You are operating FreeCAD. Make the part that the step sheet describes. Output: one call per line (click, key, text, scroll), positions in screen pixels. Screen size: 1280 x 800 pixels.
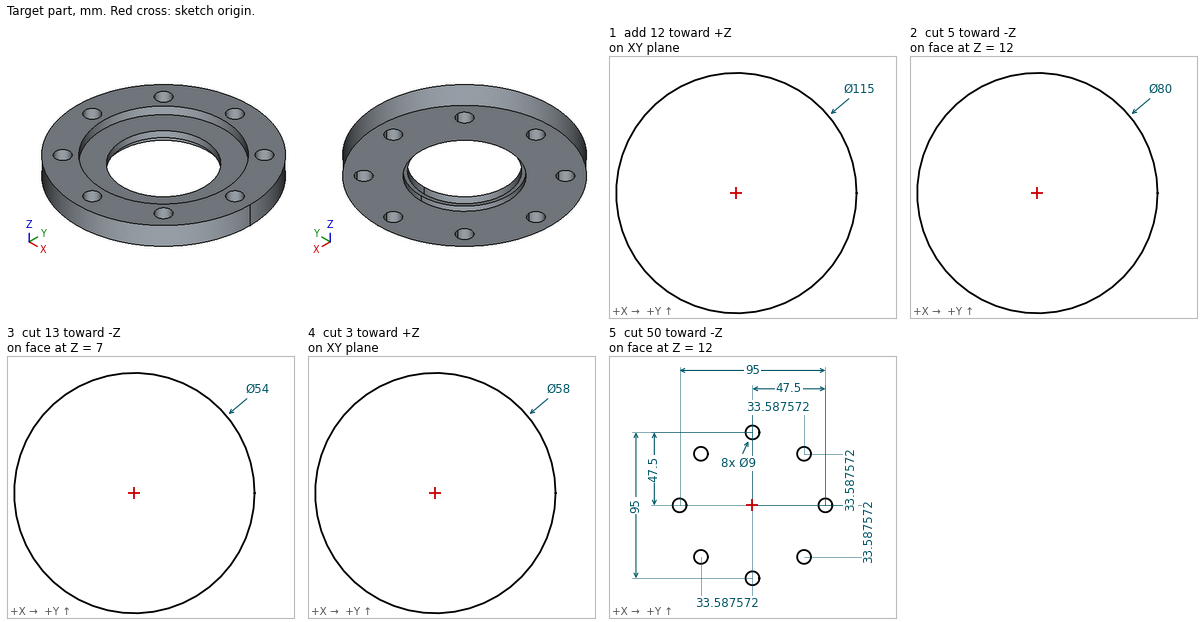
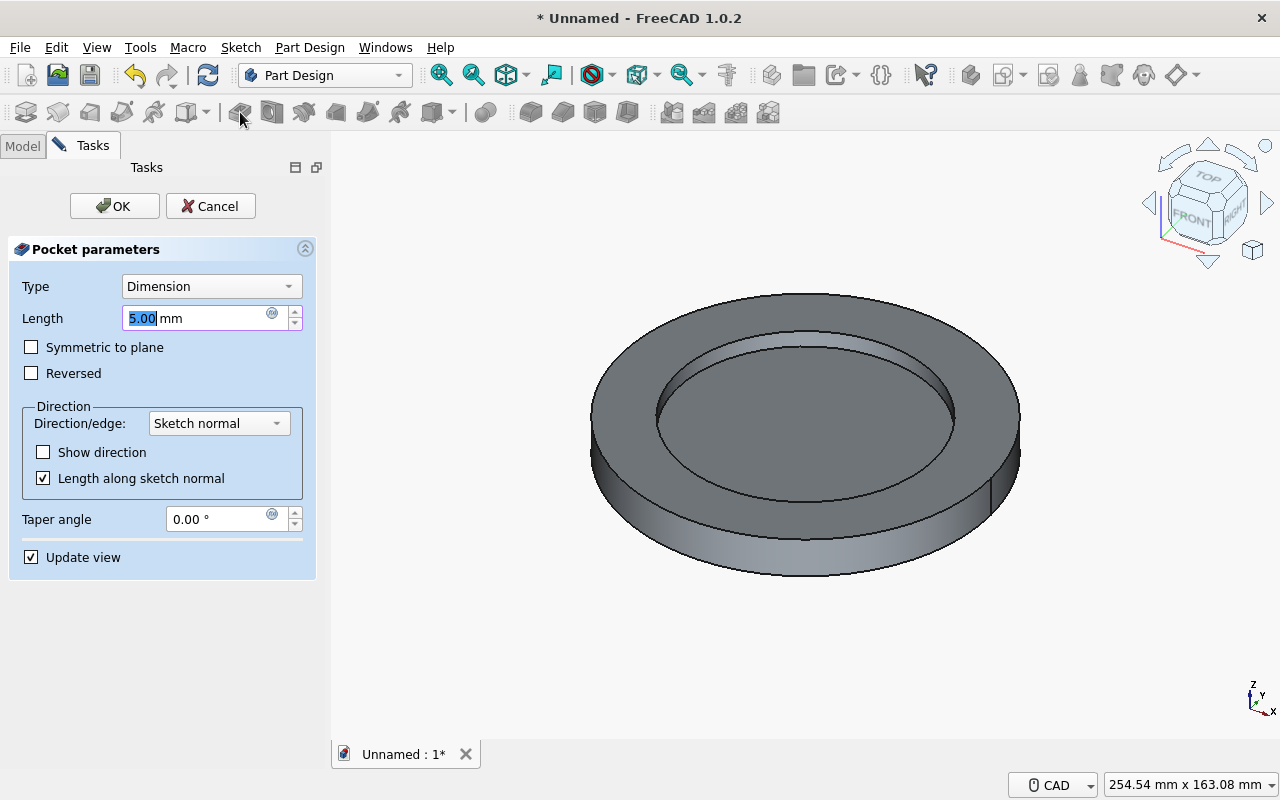
text(5)
key(Tab)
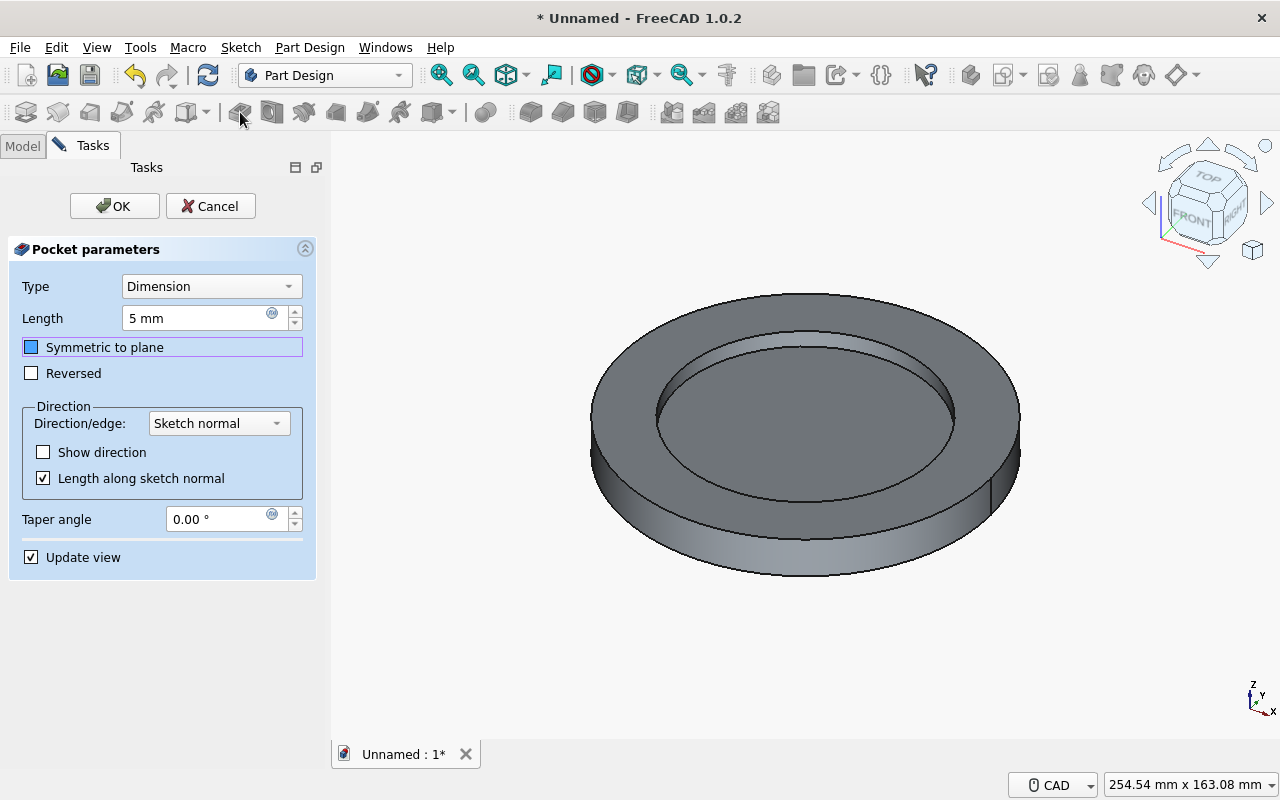
click(115, 206)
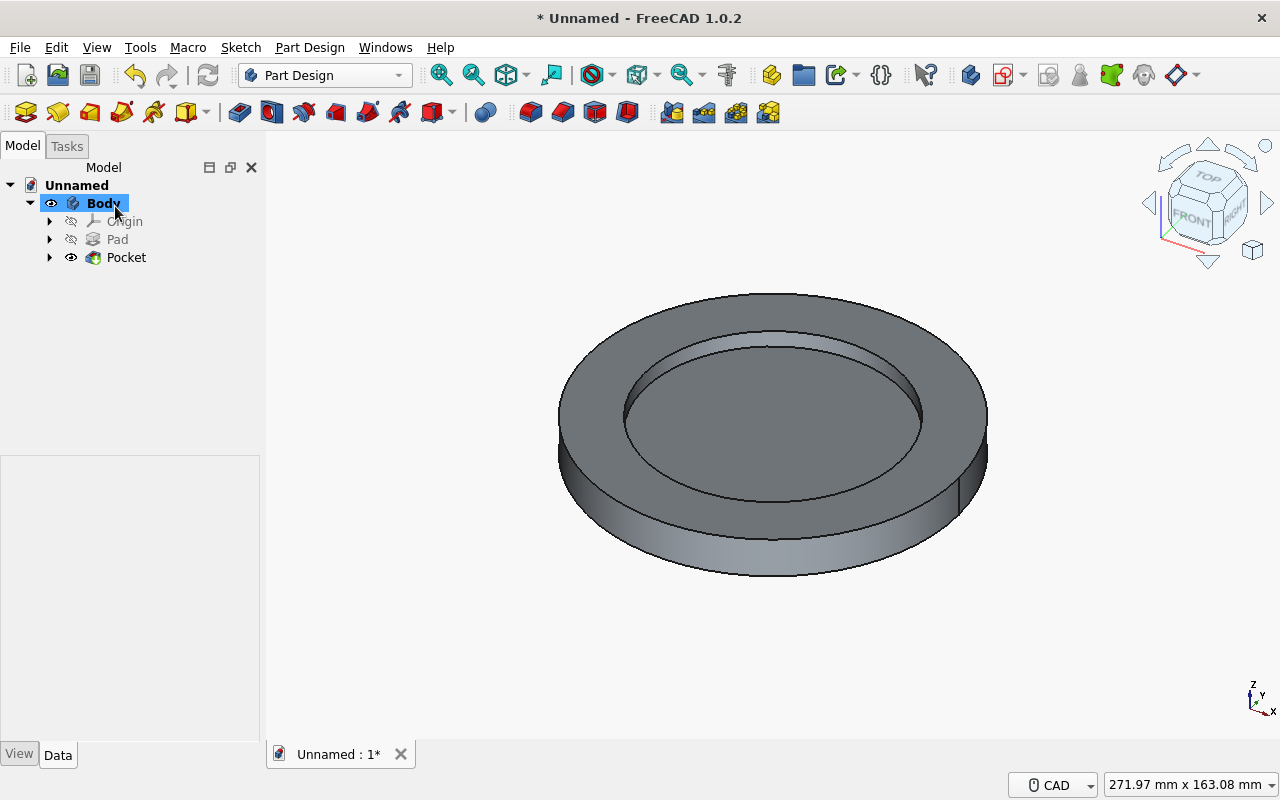
click(773, 431)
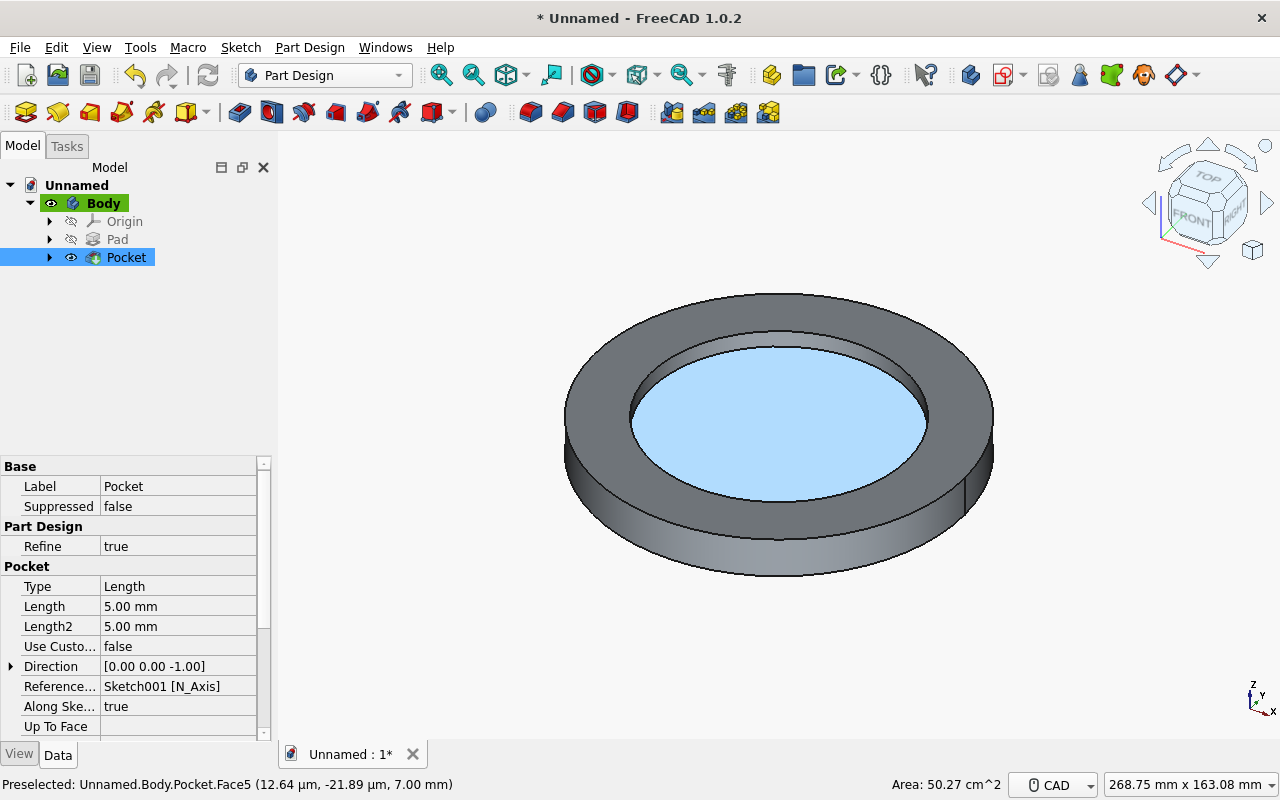
click(1004, 76)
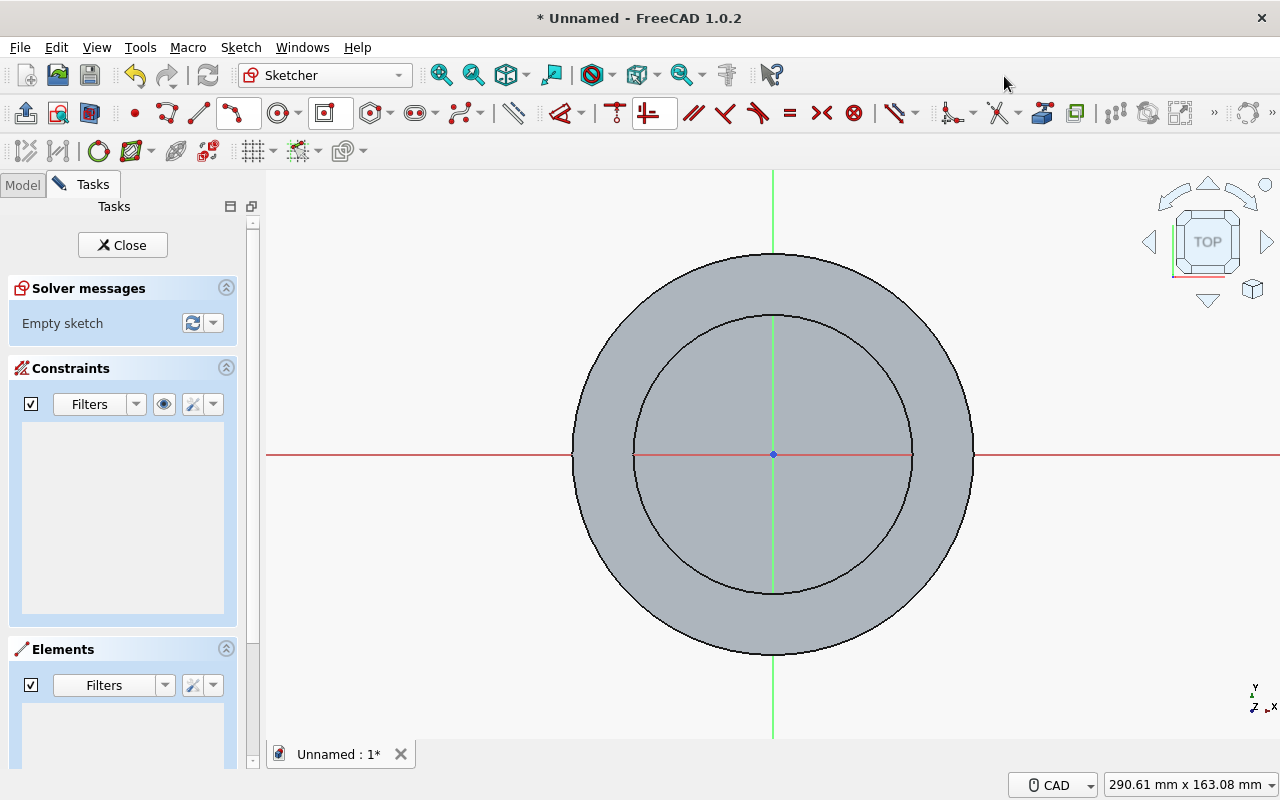
click(90, 114)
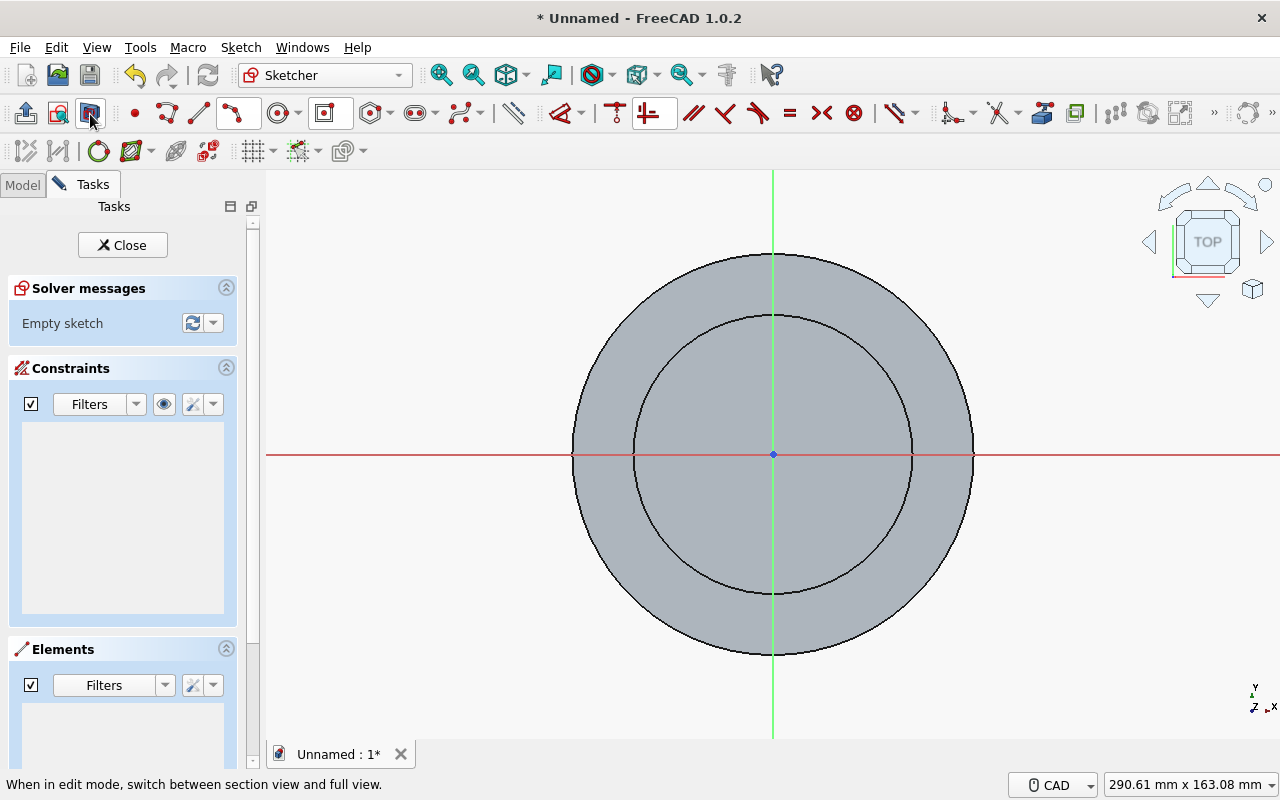
scroll(856, 454, up, 3)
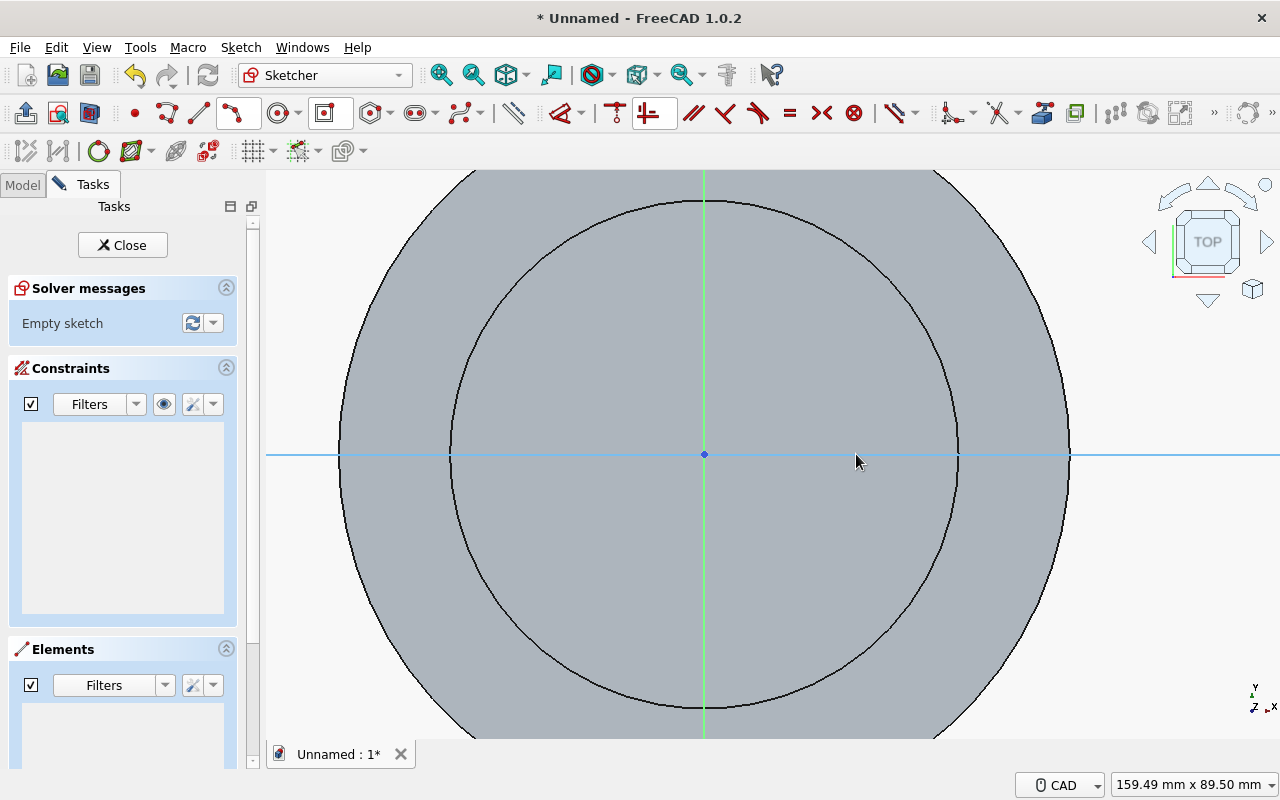
click(278, 114)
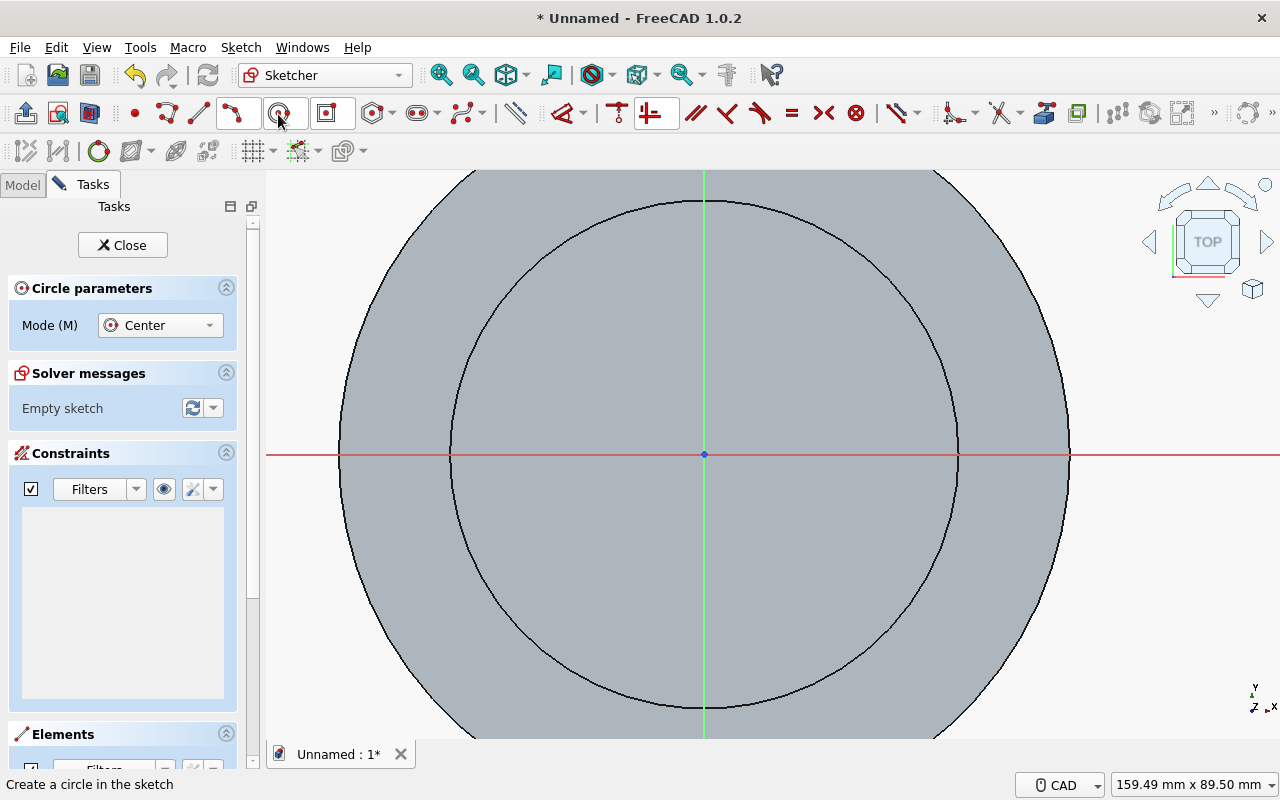
click(704, 454)
move(826, 333)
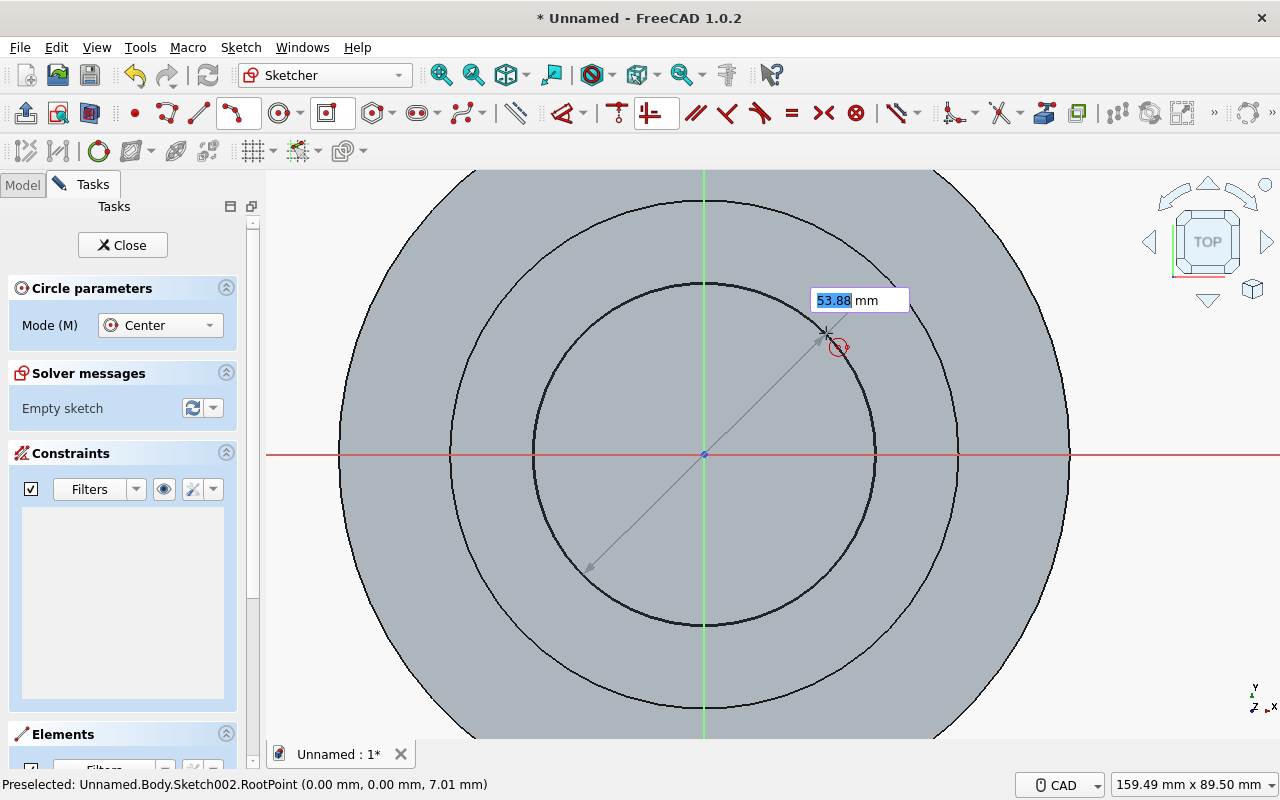
text(54)
key(Return)
key(Escape)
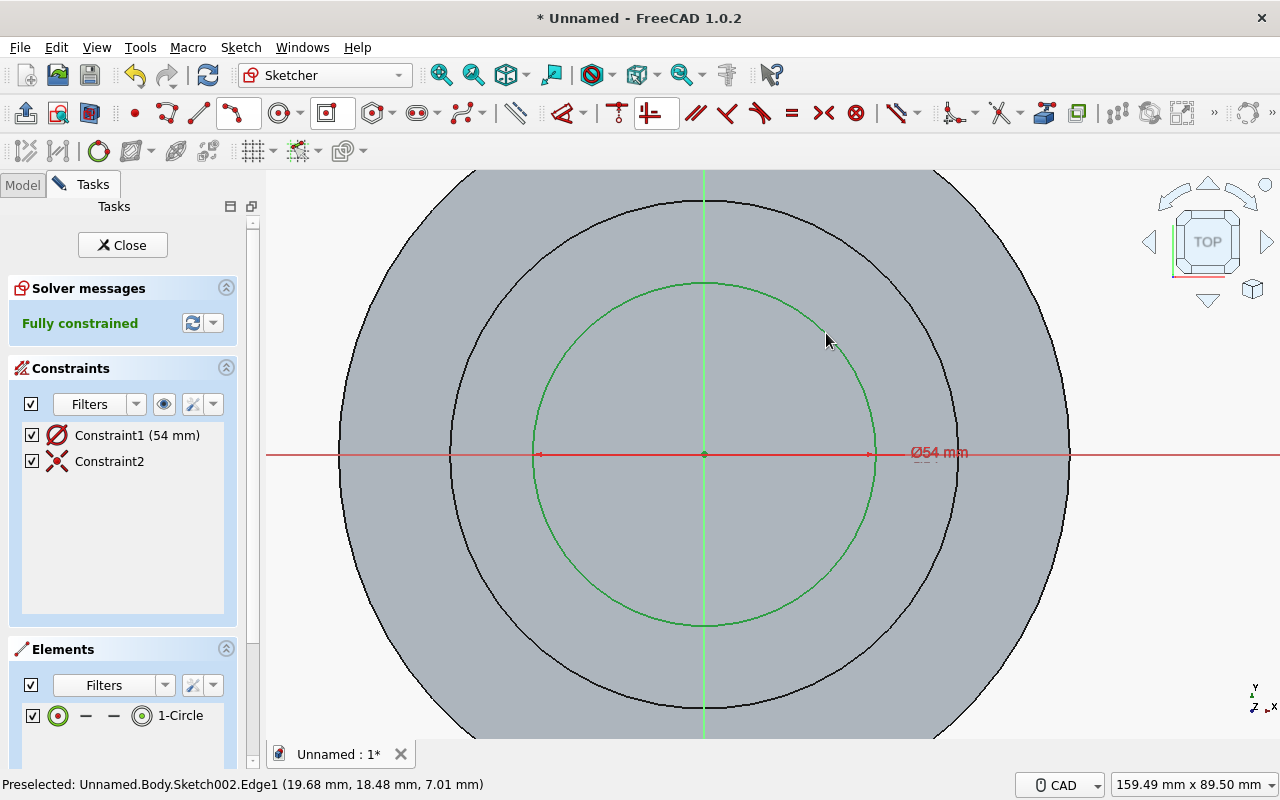
click(123, 245)